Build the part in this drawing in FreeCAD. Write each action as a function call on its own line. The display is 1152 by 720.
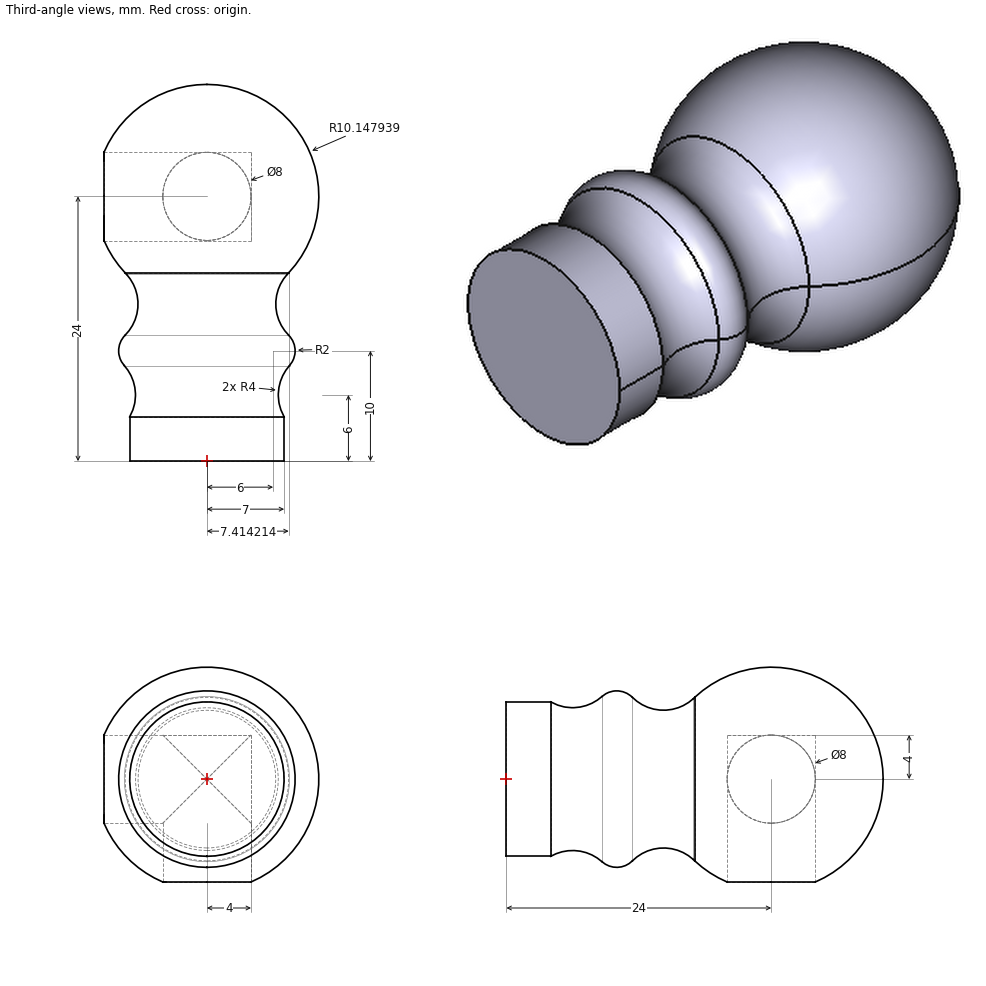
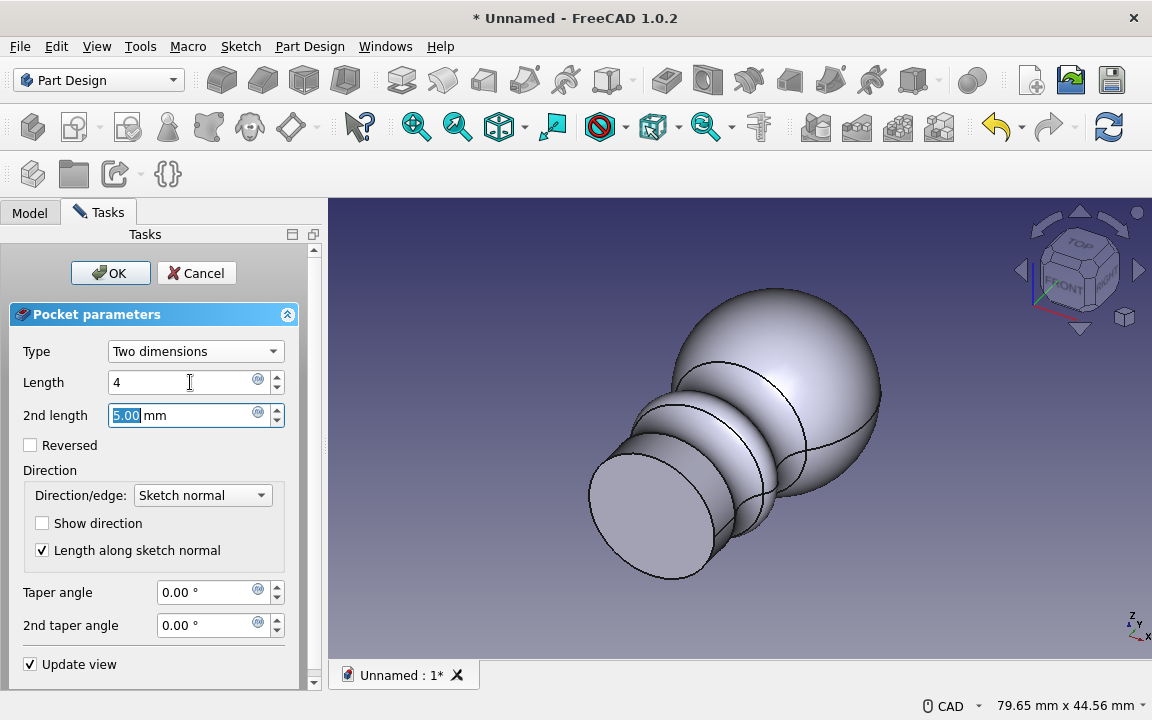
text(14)
key(Tab)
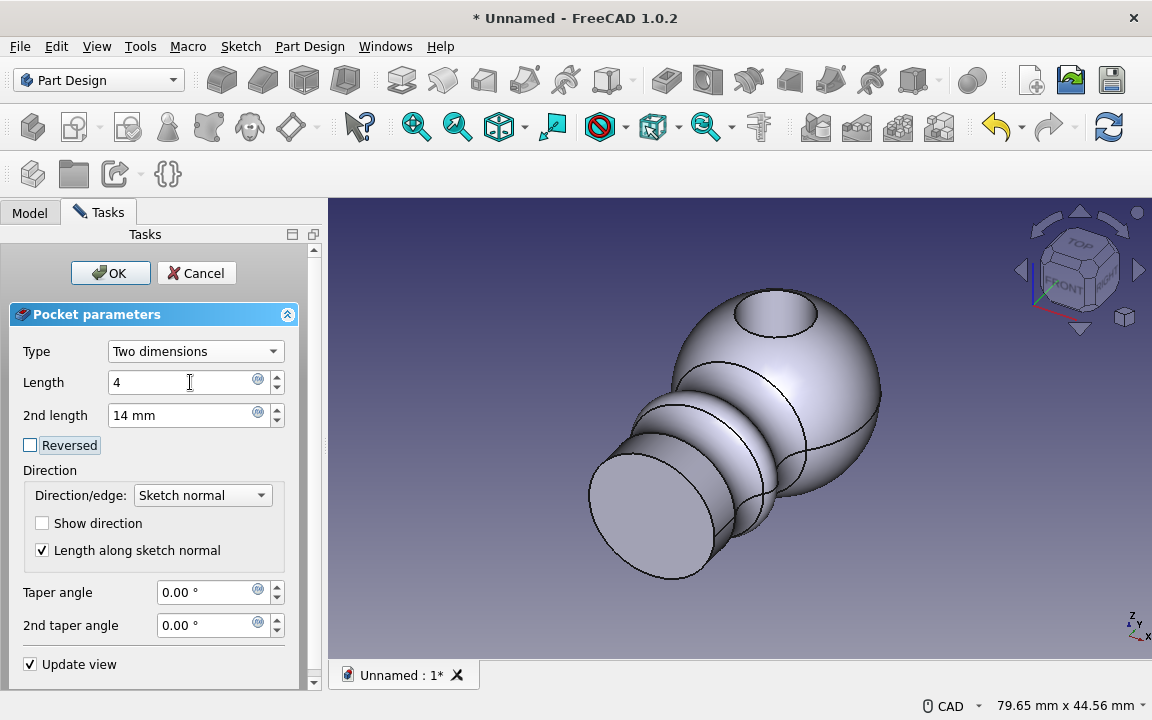
click(31, 445)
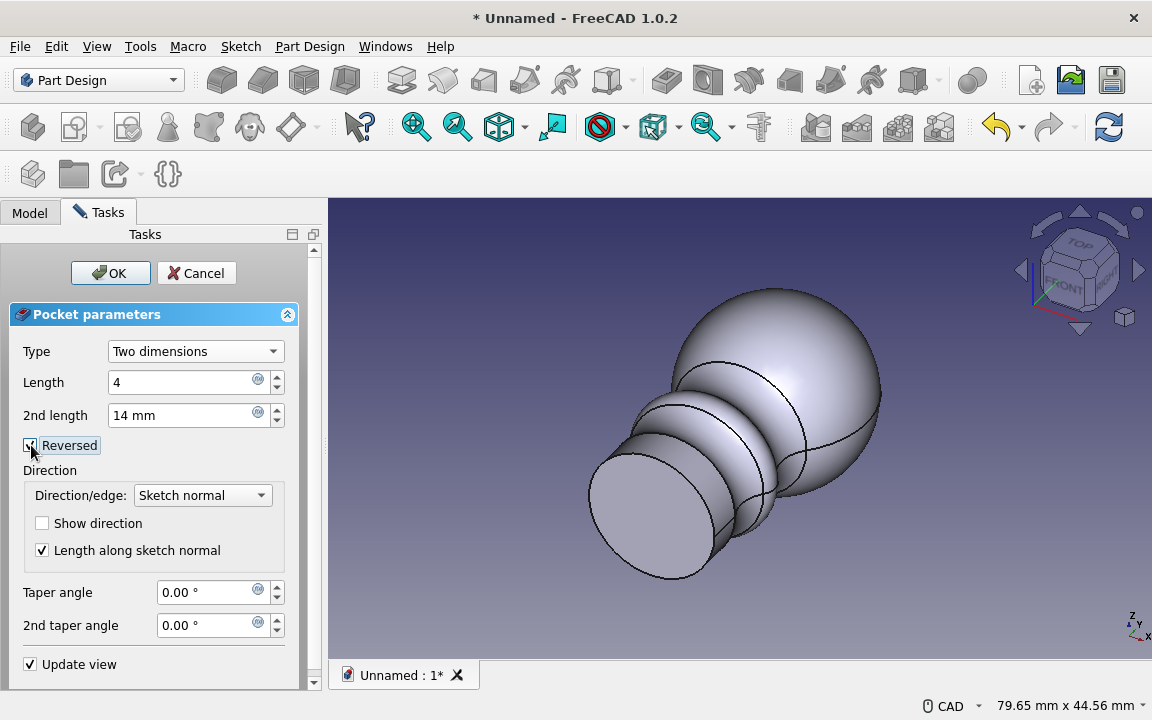
click(111, 273)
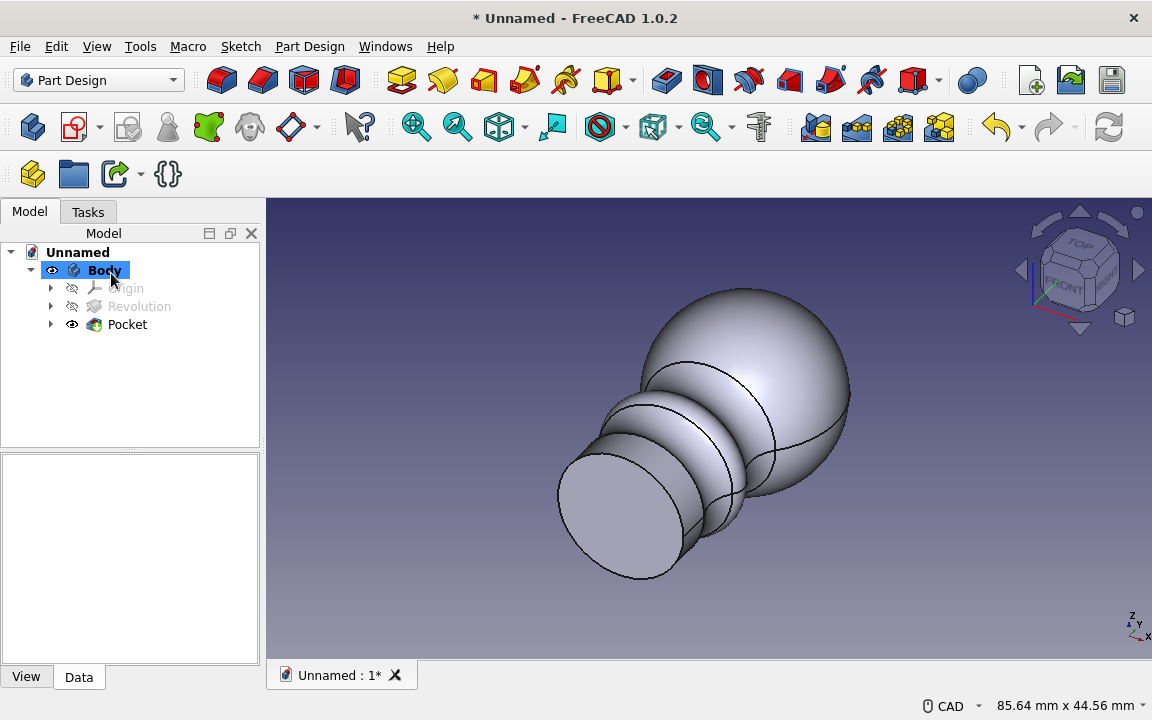
click(74, 128)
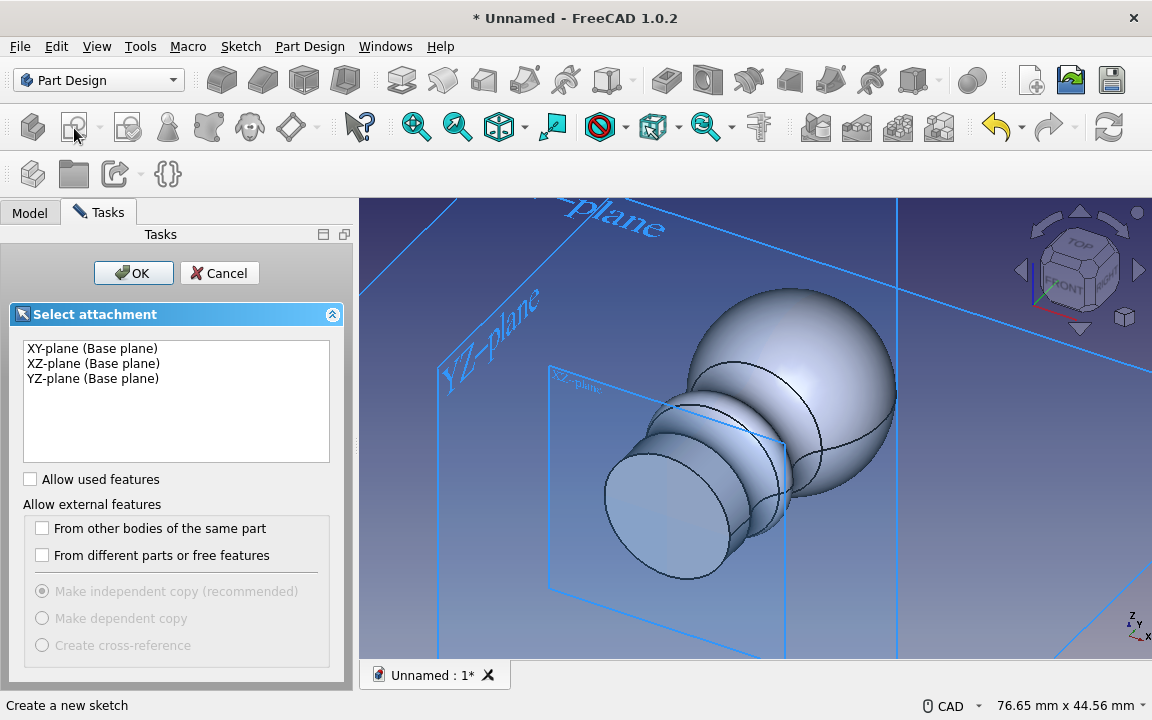
click(84, 378)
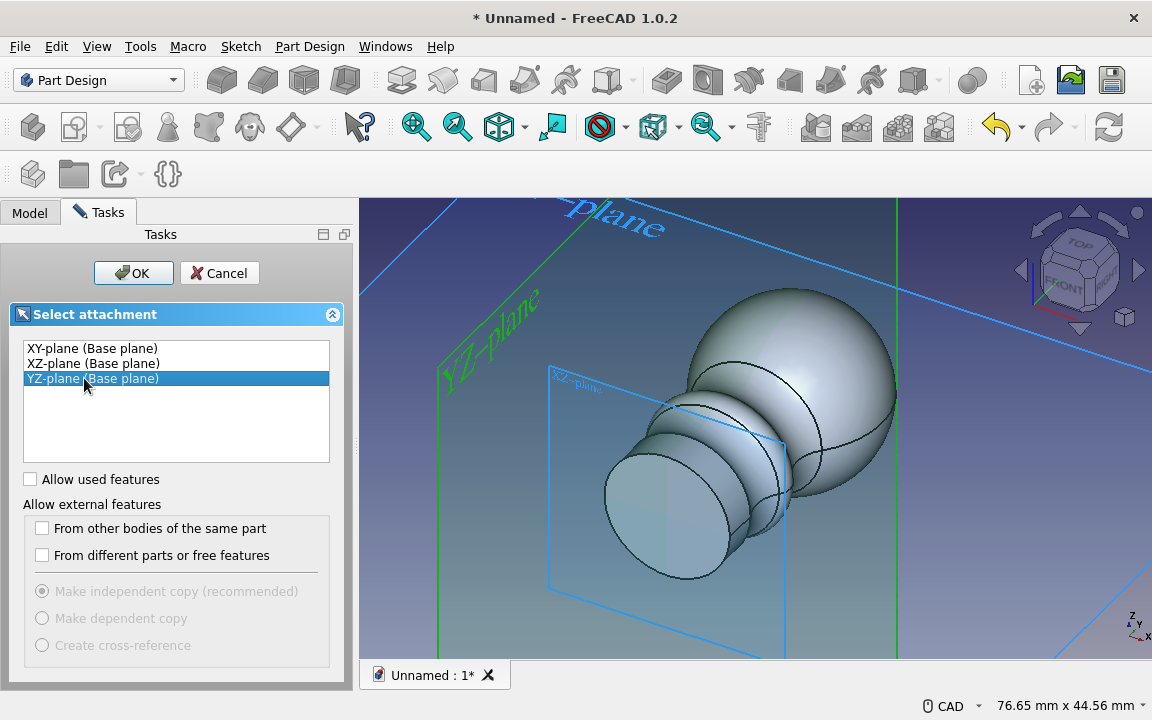
click(134, 273)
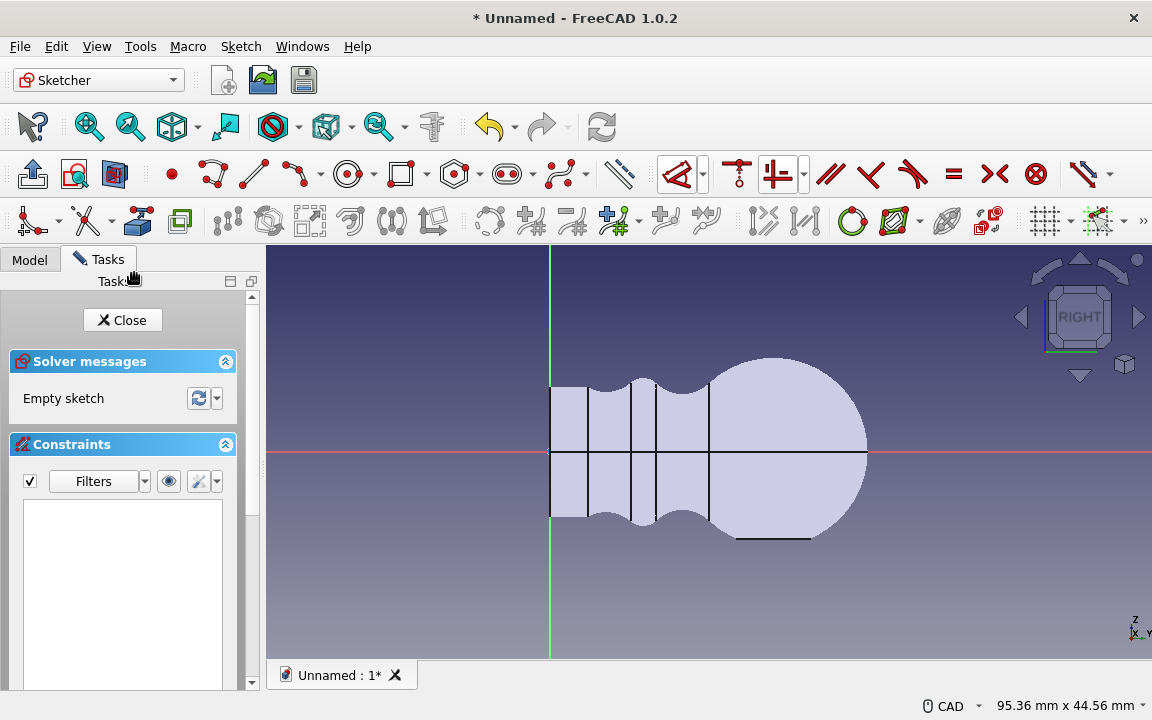
click(115, 174)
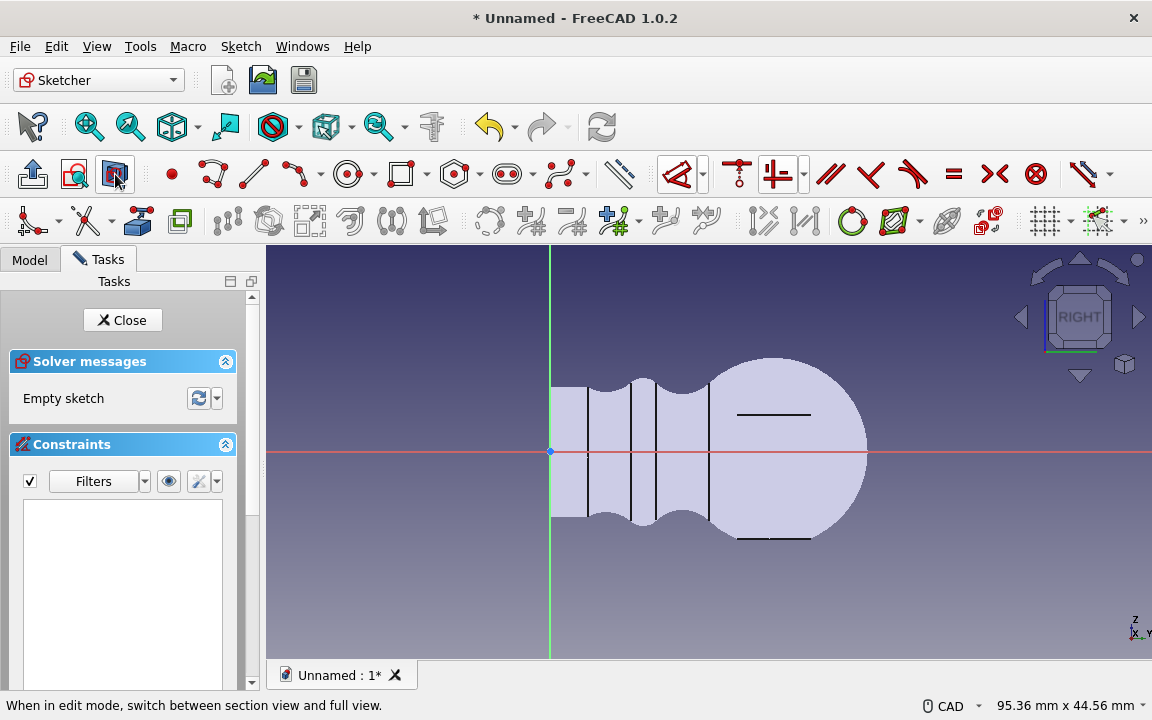
scroll(831, 452, up, 6)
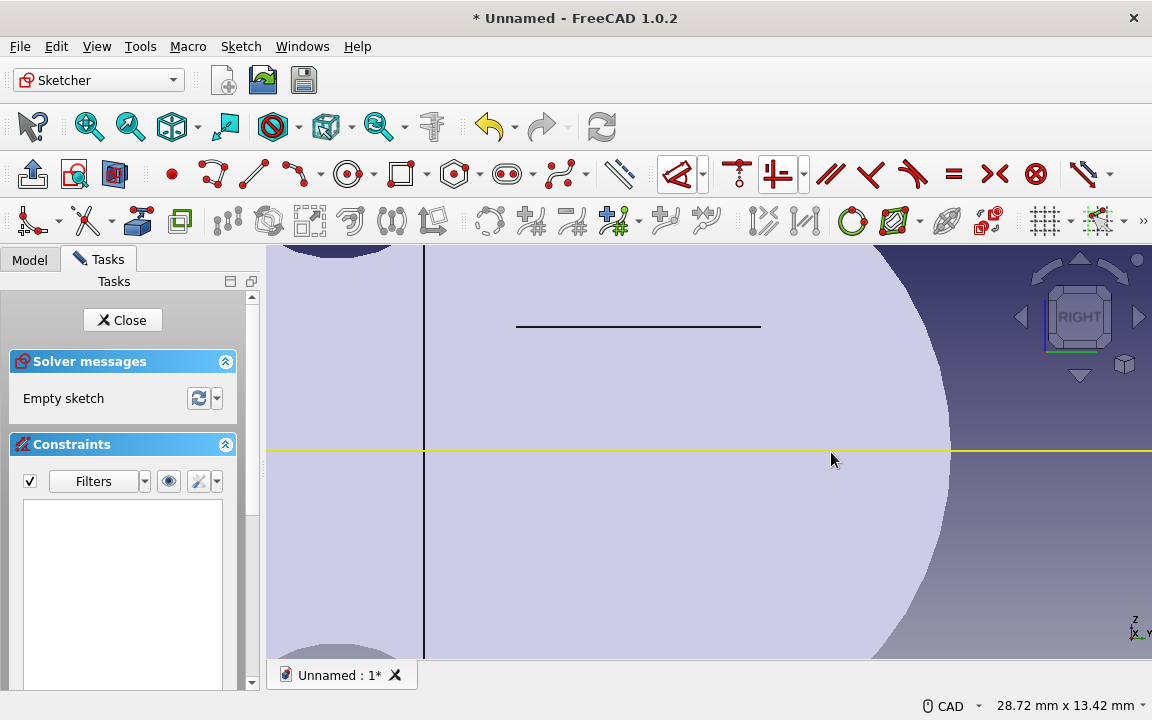
click(348, 174)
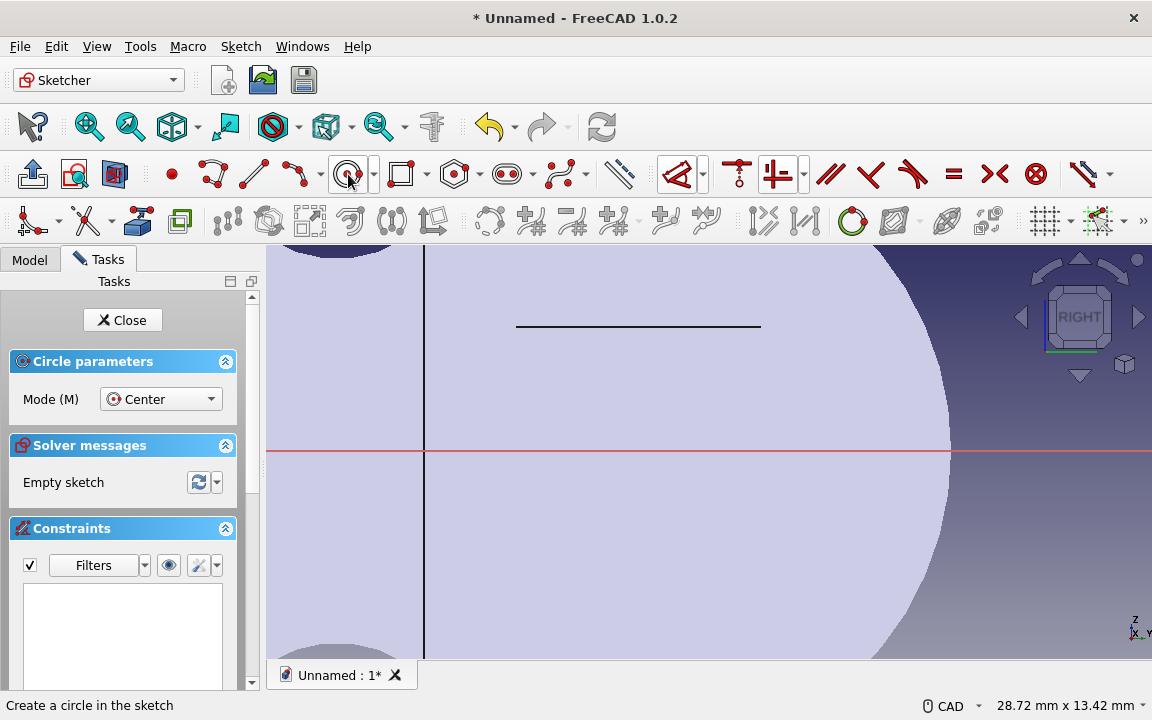
click(638, 451)
click(725, 364)
key(Escape)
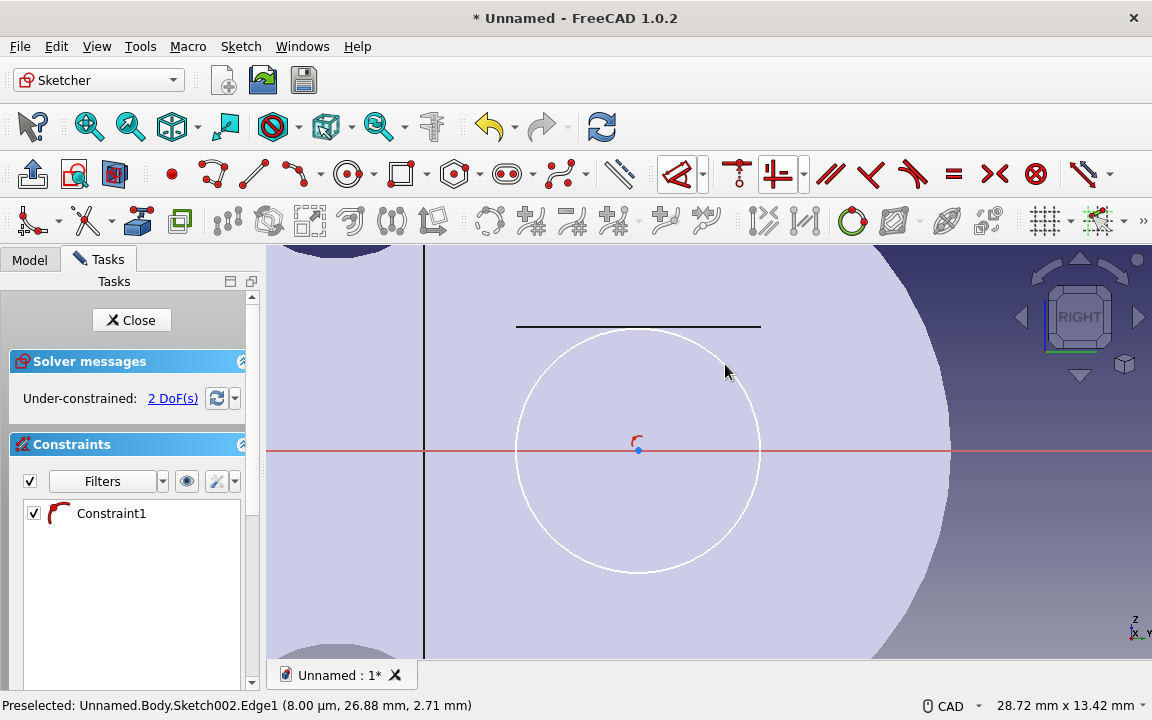
click(724, 364)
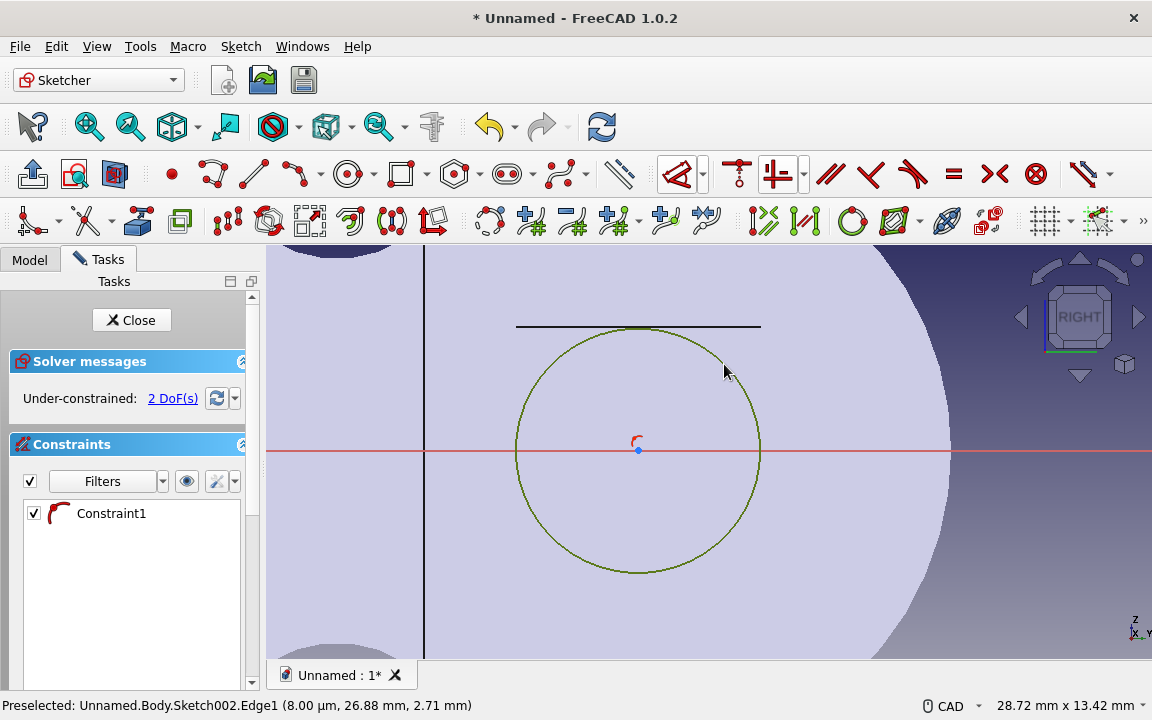
key(k)
key(o)